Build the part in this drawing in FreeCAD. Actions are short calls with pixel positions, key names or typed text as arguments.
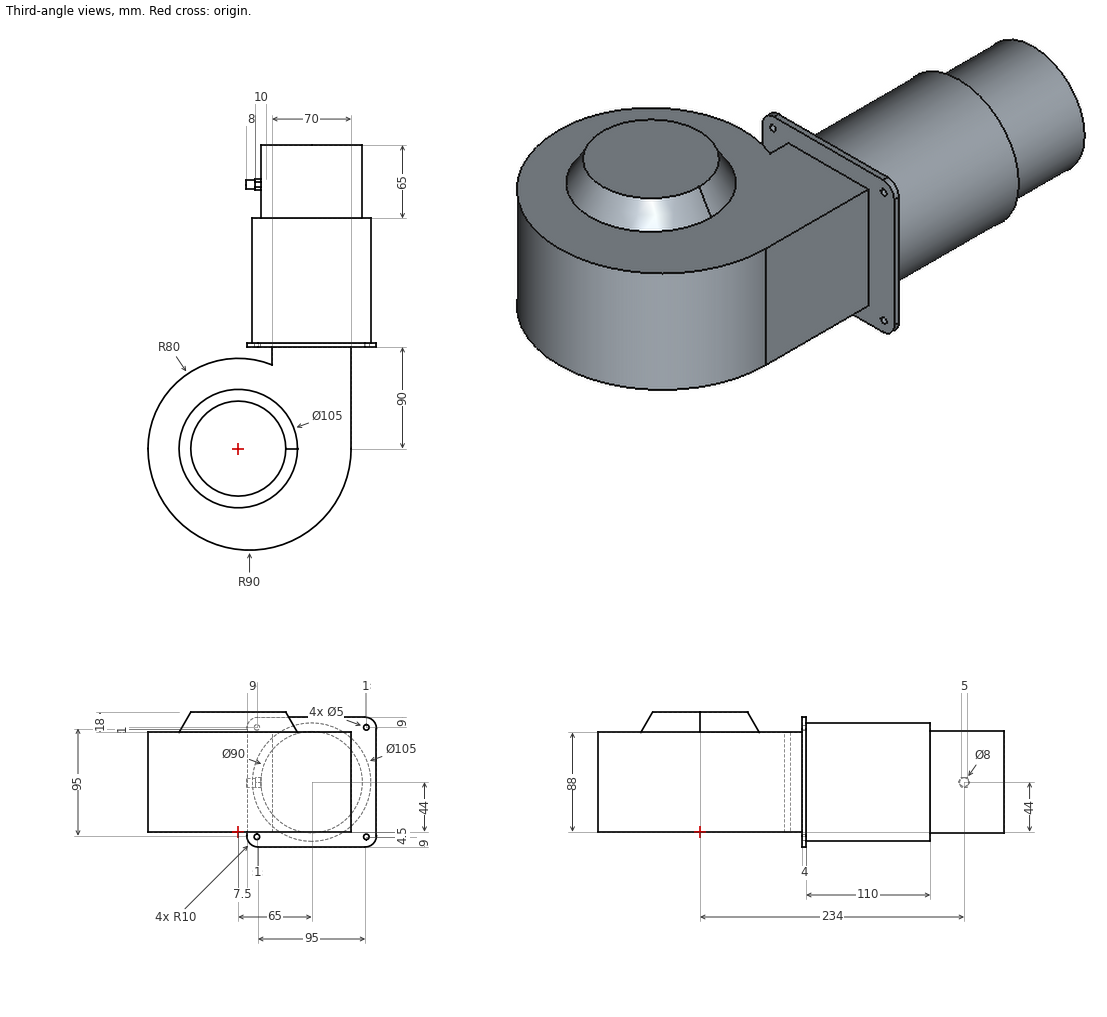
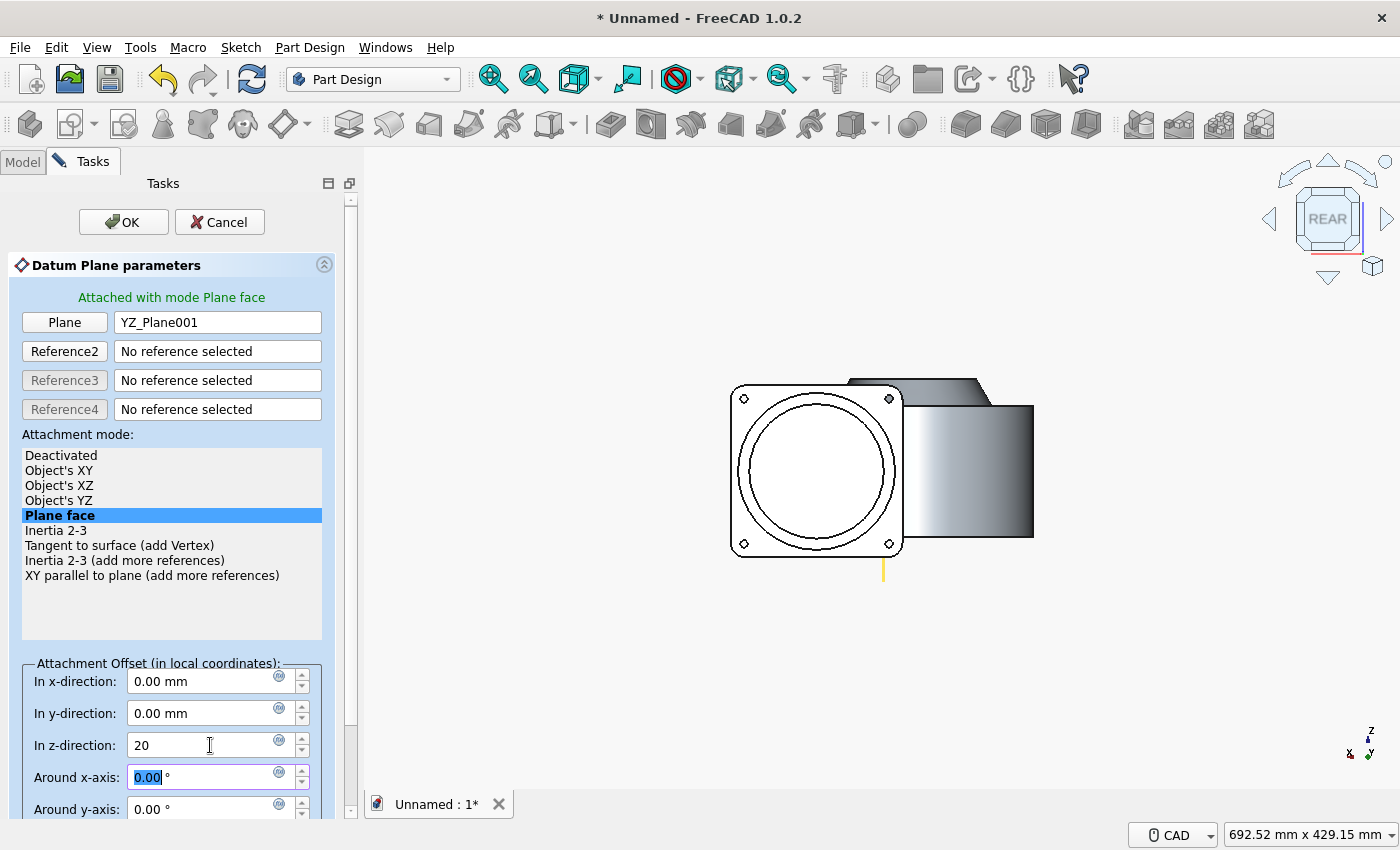
click(124, 222)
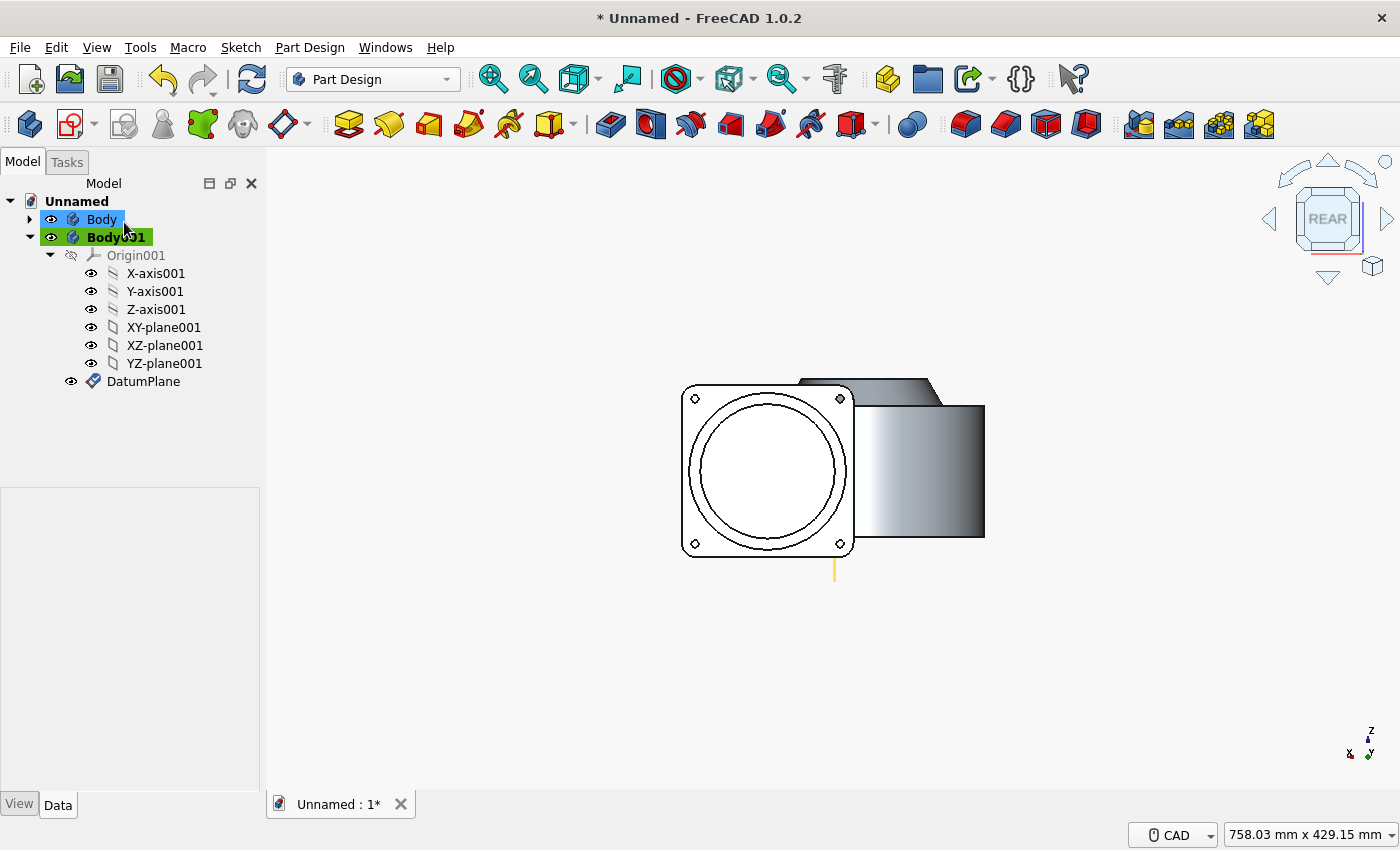
click(116, 381)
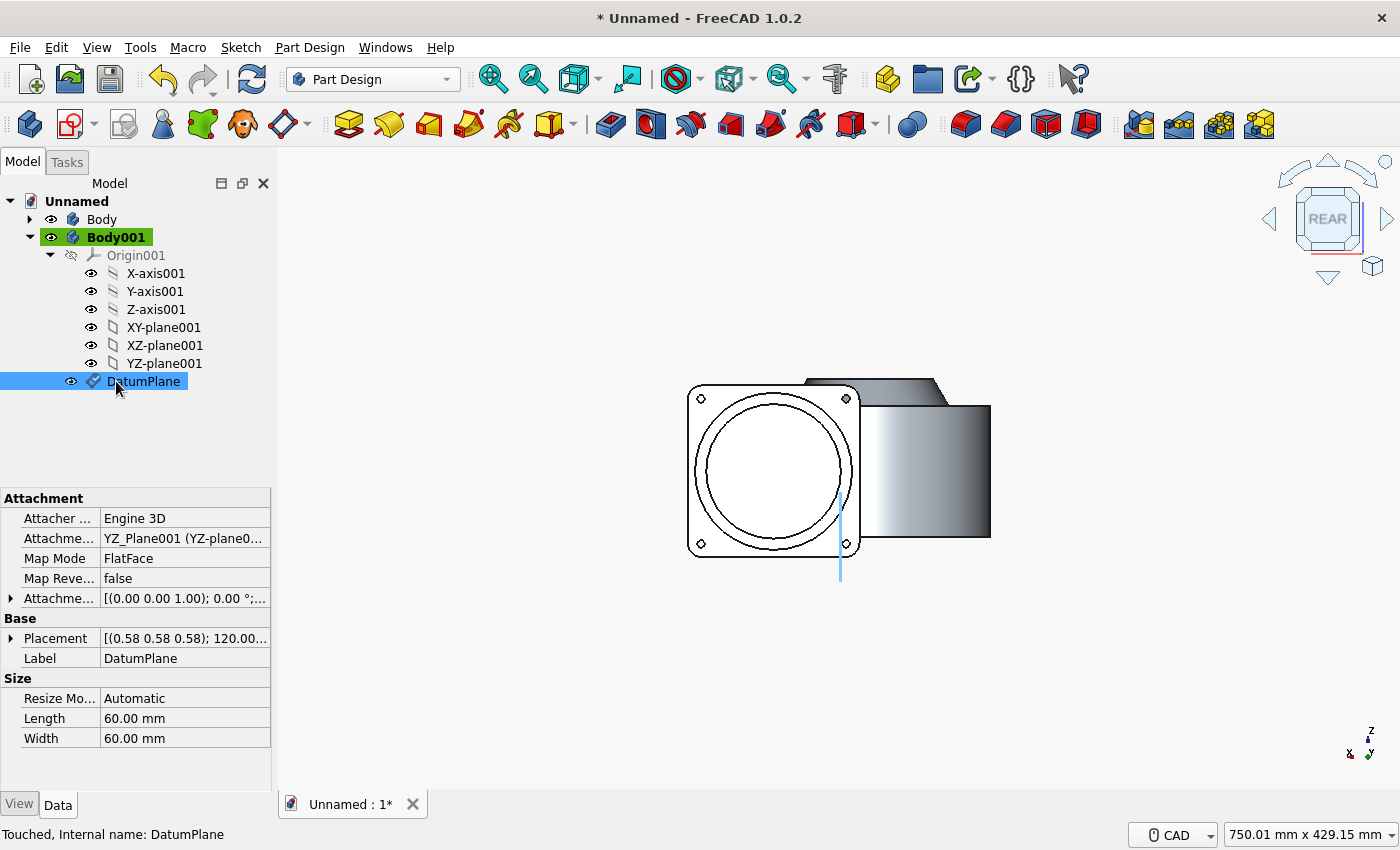
click(70, 124)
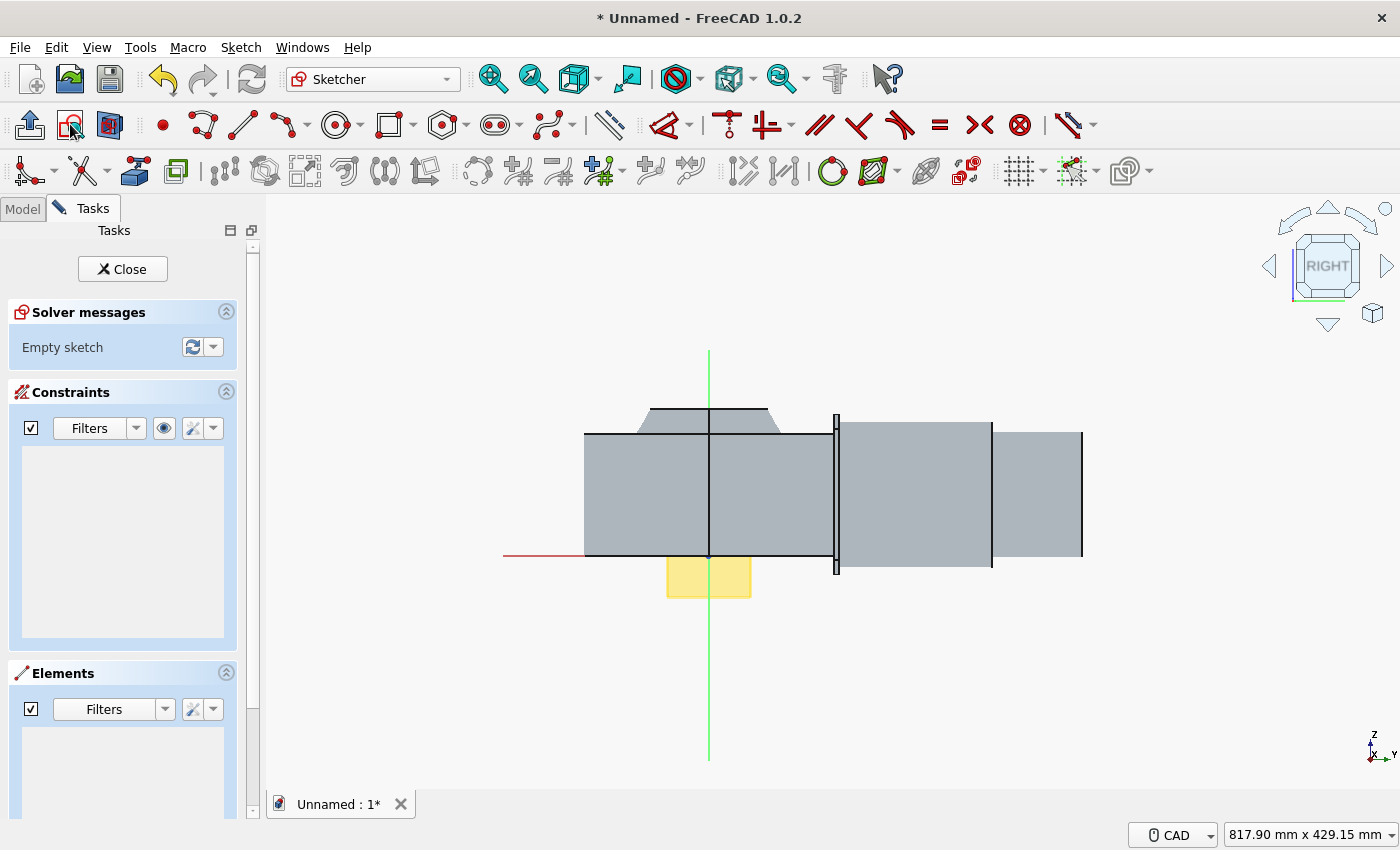
scroll(1047, 495, up, 15)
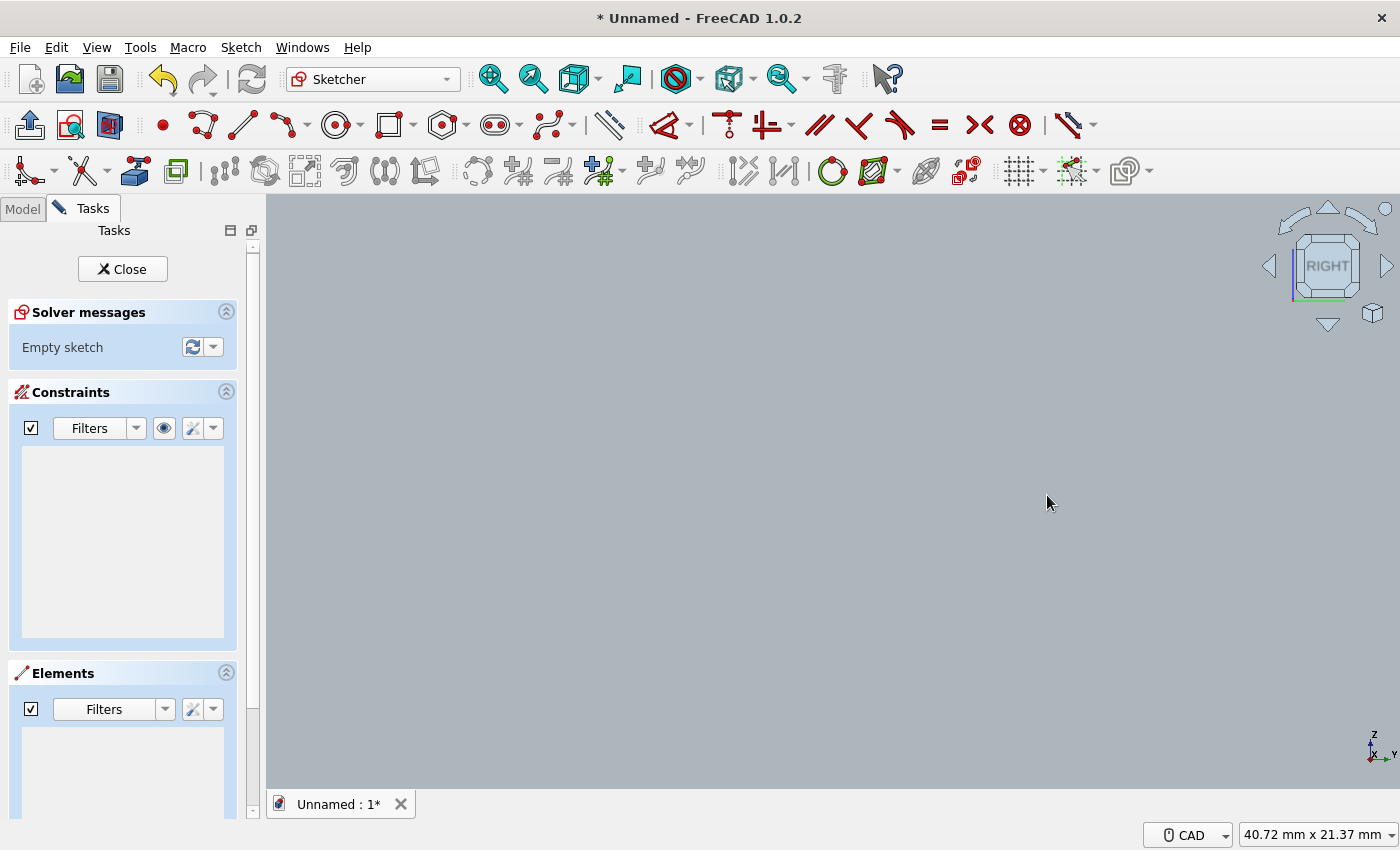
scroll(750, 450, up, 2)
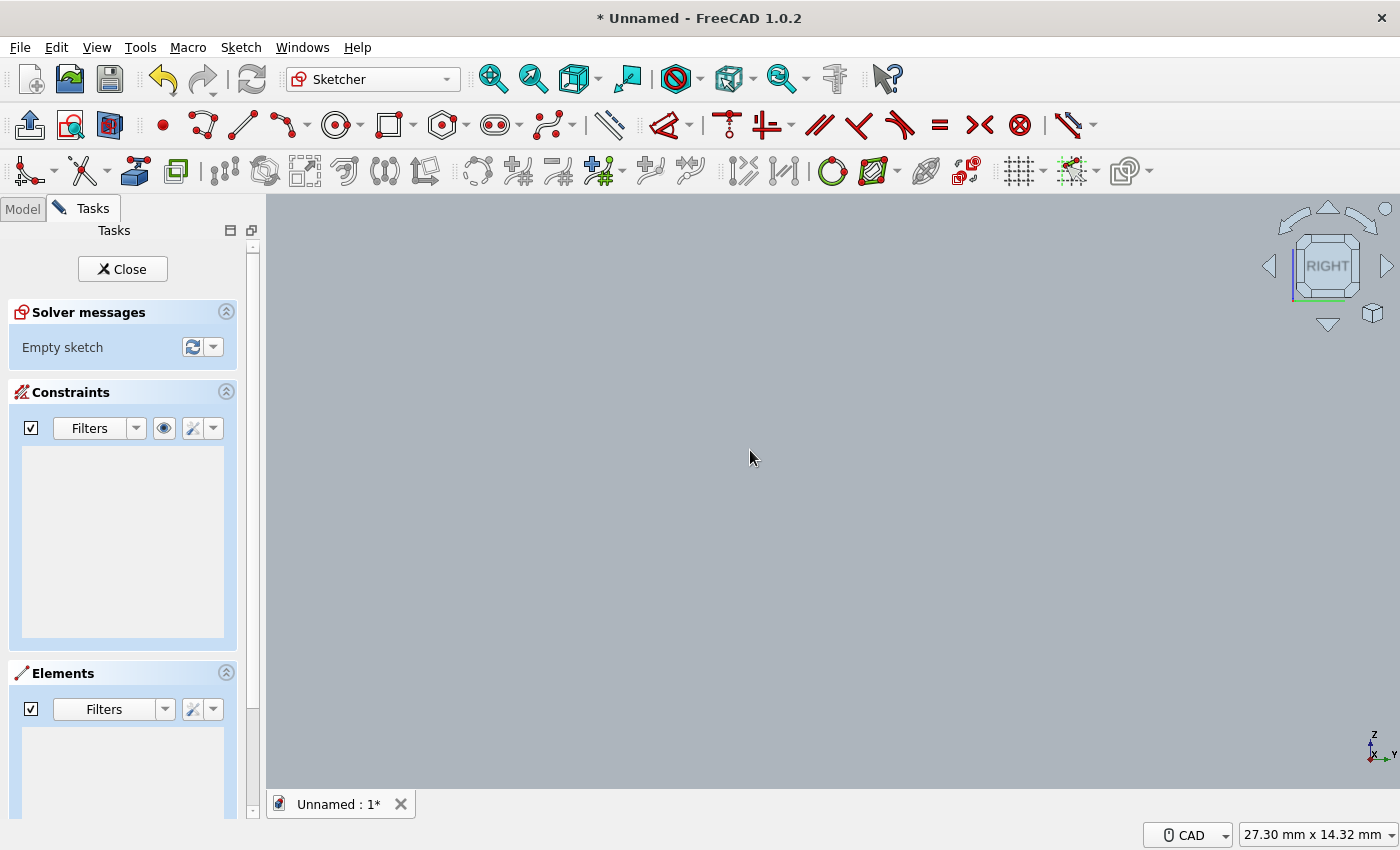
click(442, 126)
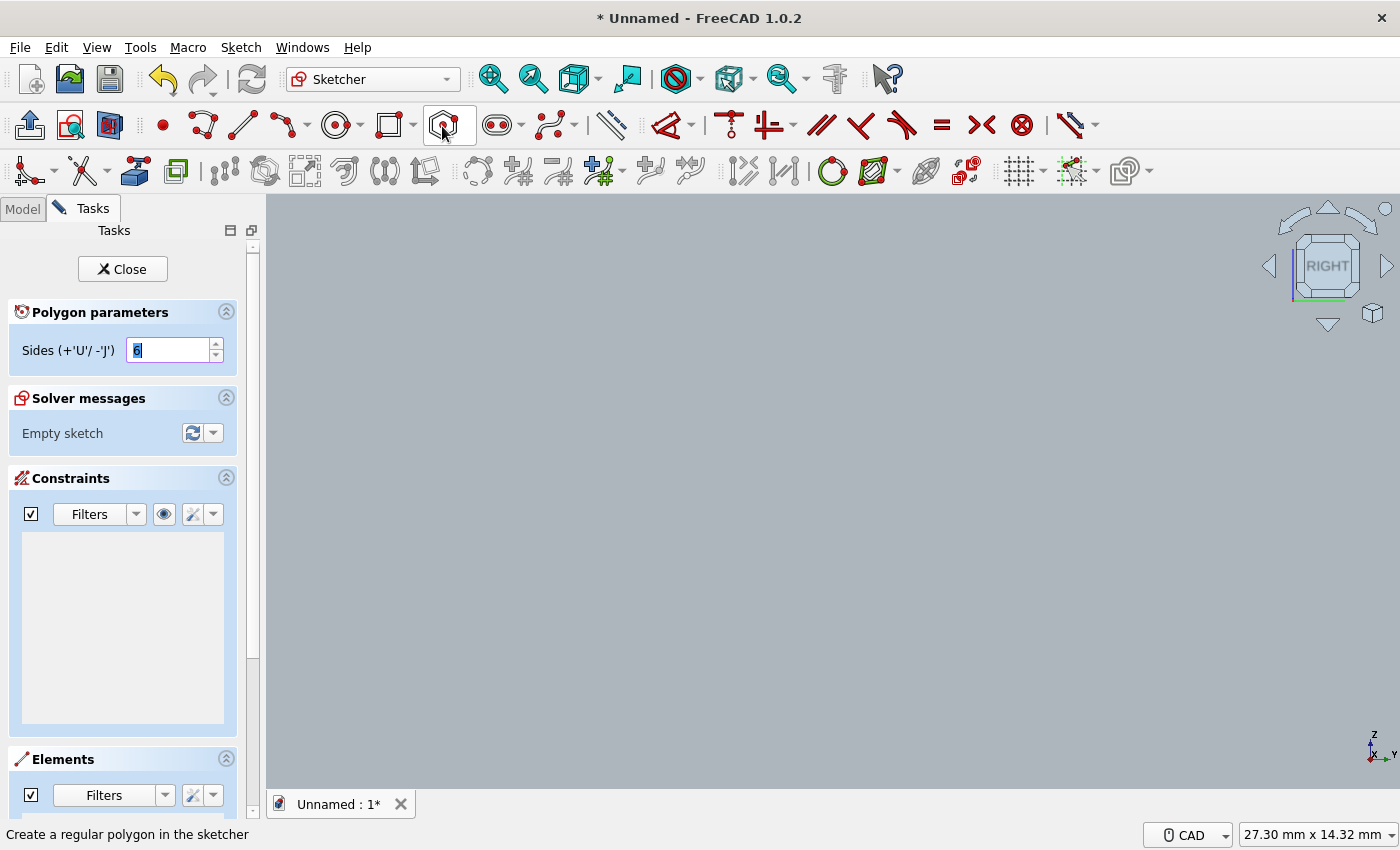
click(764, 491)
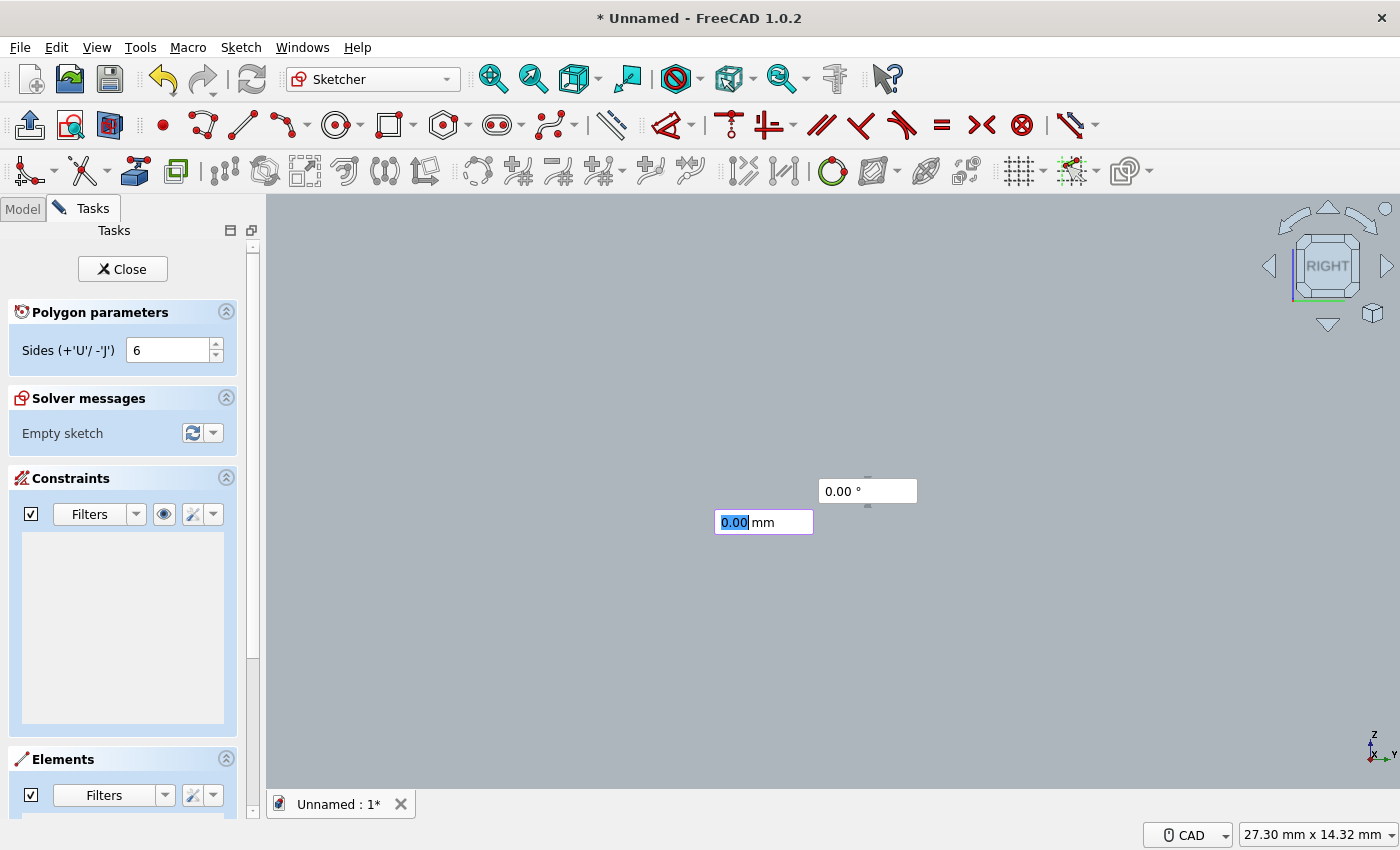
click(972, 491)
key(Escape)